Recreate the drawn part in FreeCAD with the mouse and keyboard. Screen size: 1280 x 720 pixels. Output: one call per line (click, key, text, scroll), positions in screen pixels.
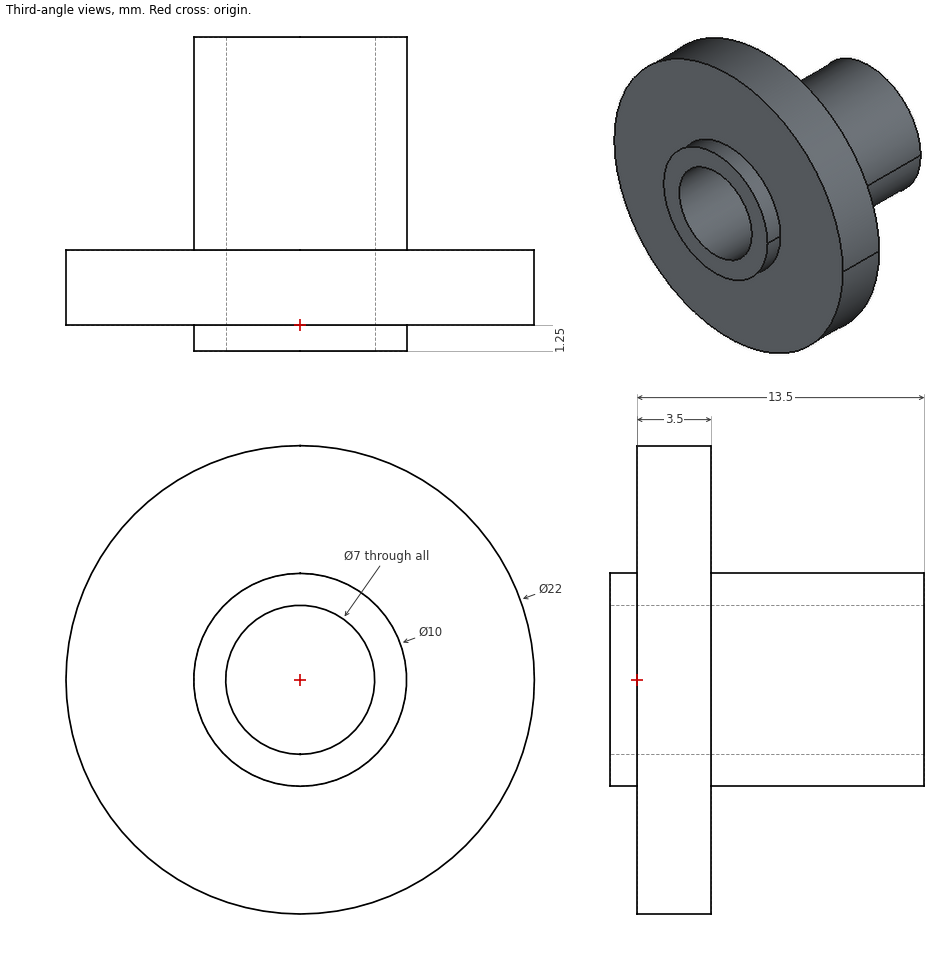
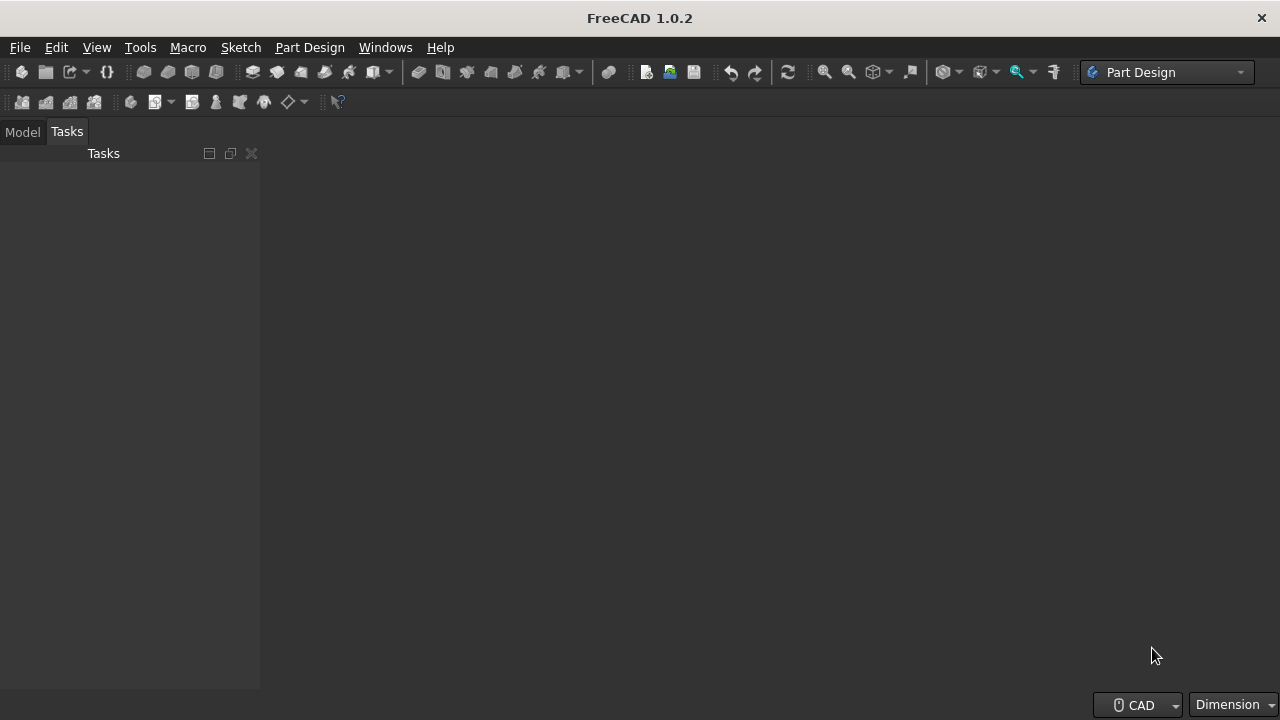
click(646, 72)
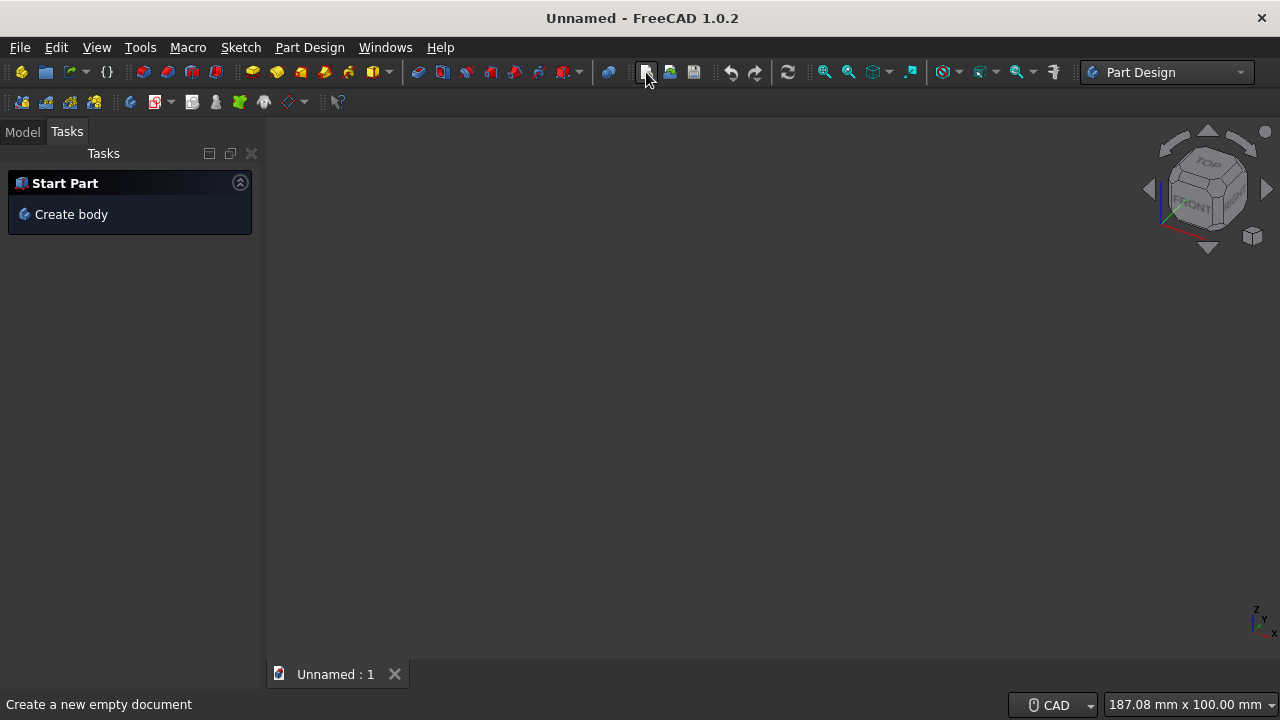
click(156, 102)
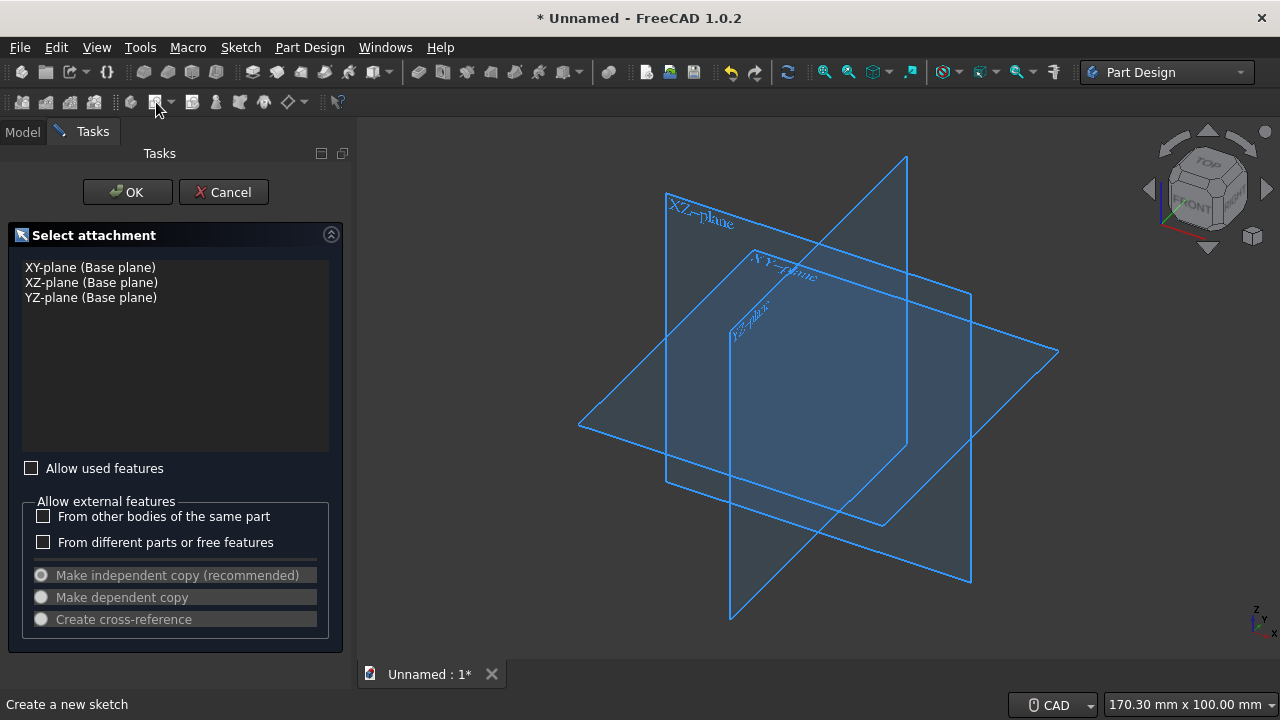
click(82, 282)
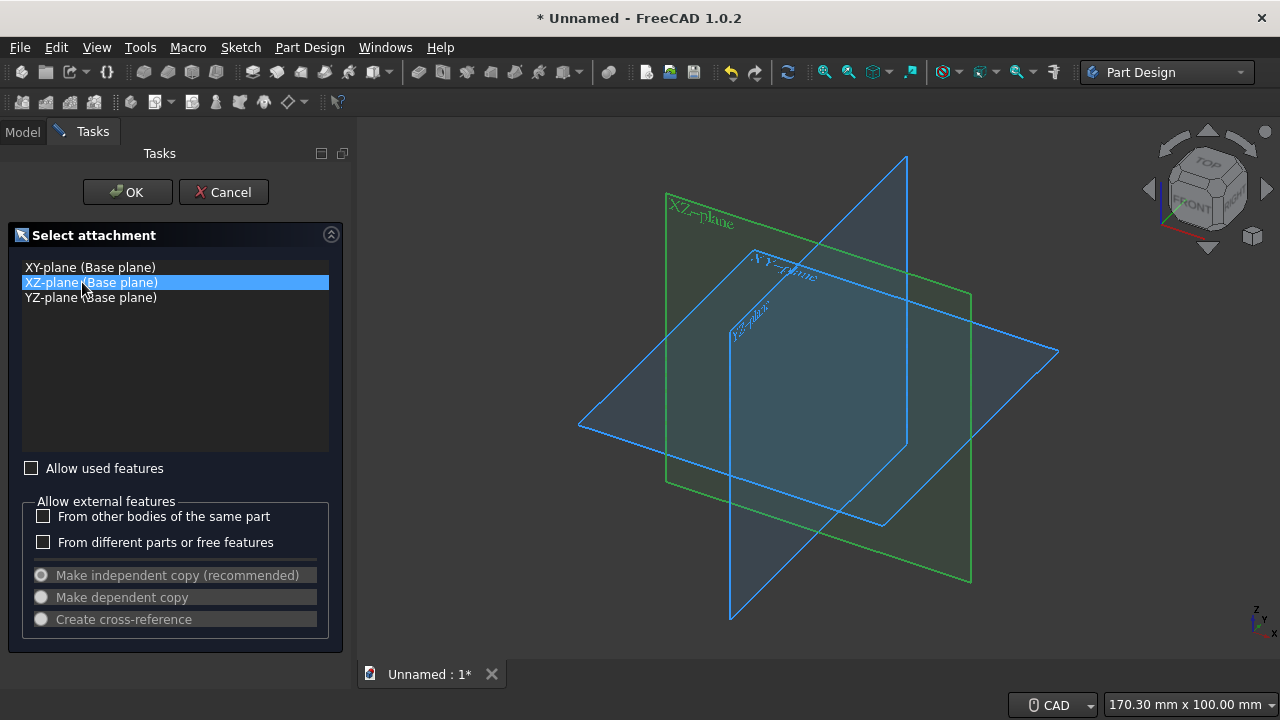
click(128, 192)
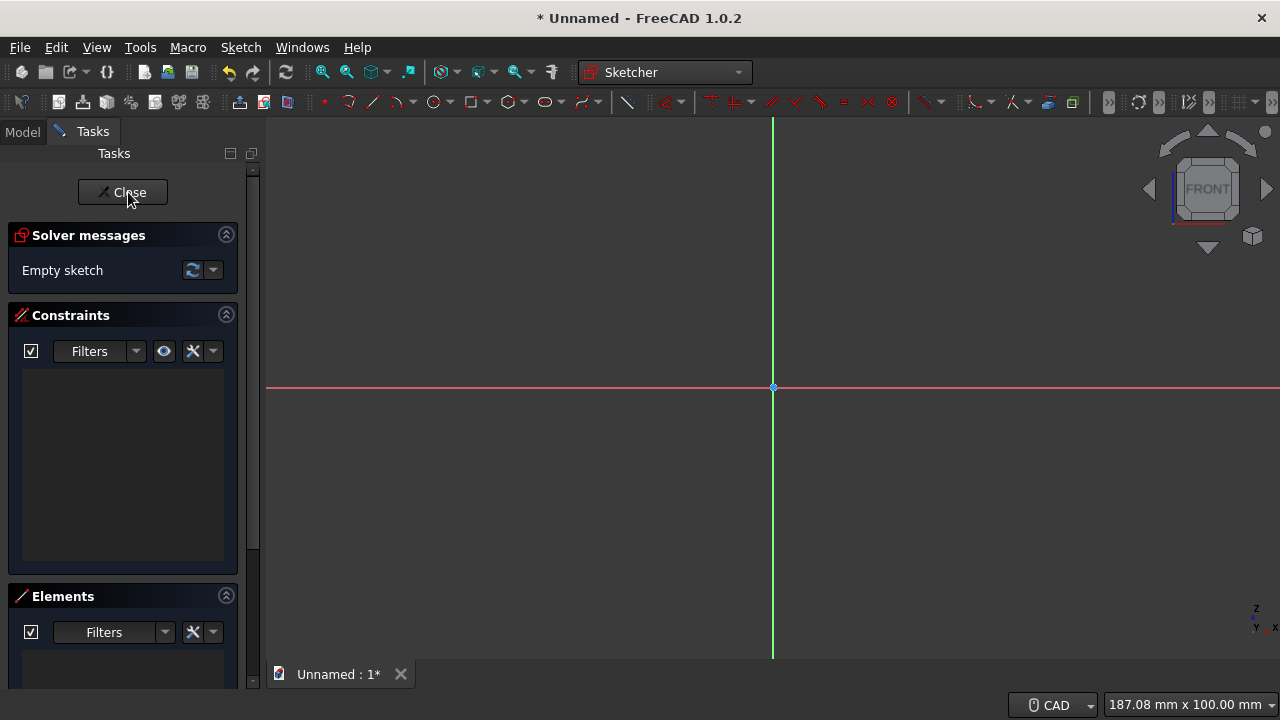
scroll(813, 388, up, 5)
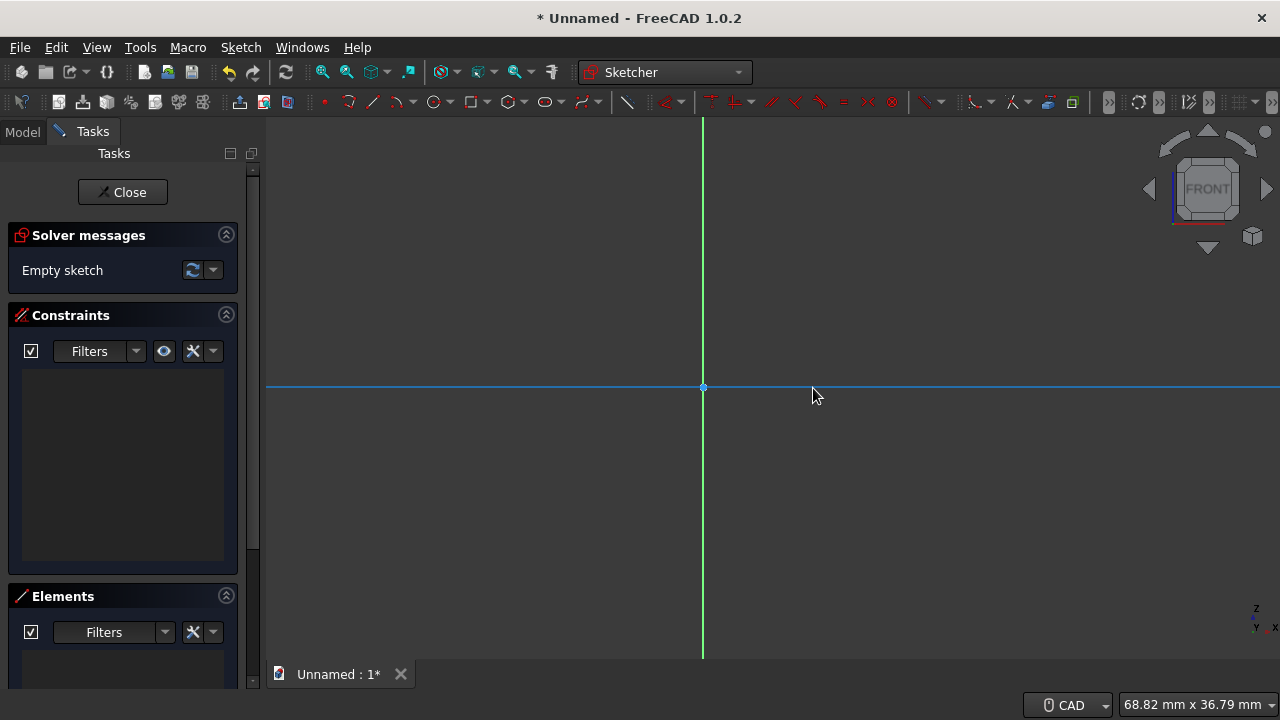
key(g)
key(c)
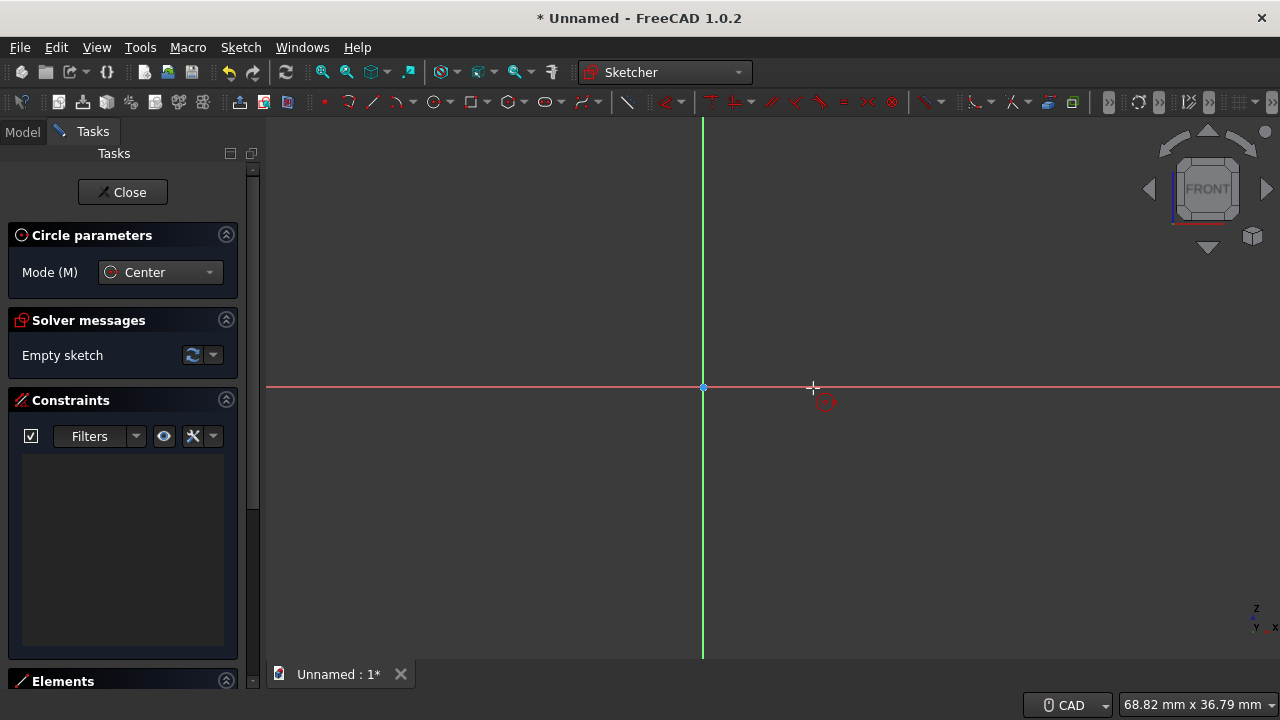
click(703, 387)
move(818, 273)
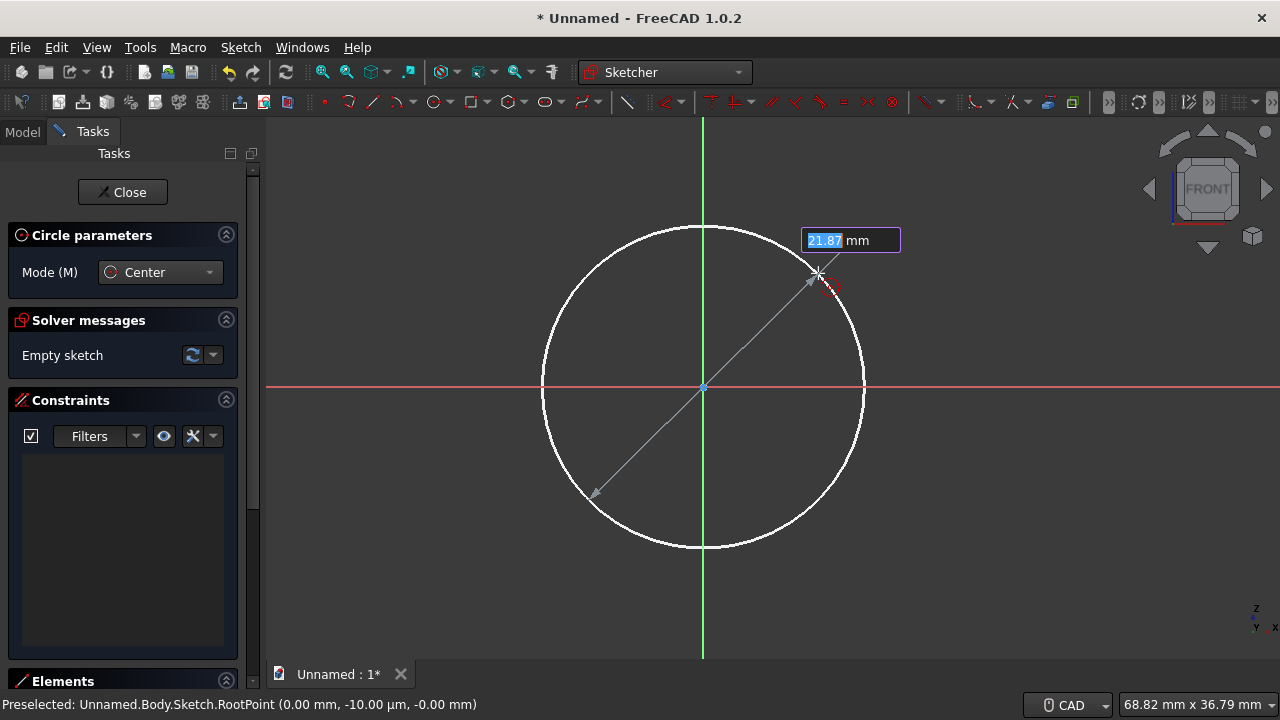
text(22)
key(Return)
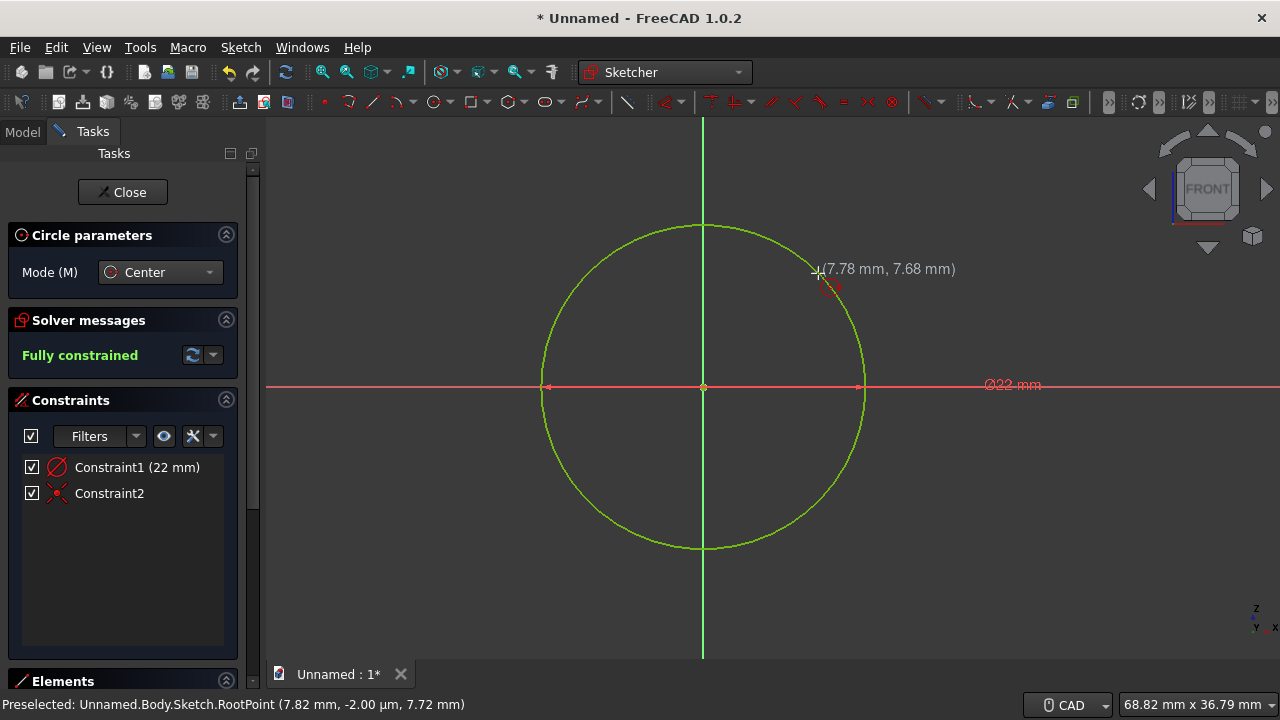
click(703, 387)
move(755, 335)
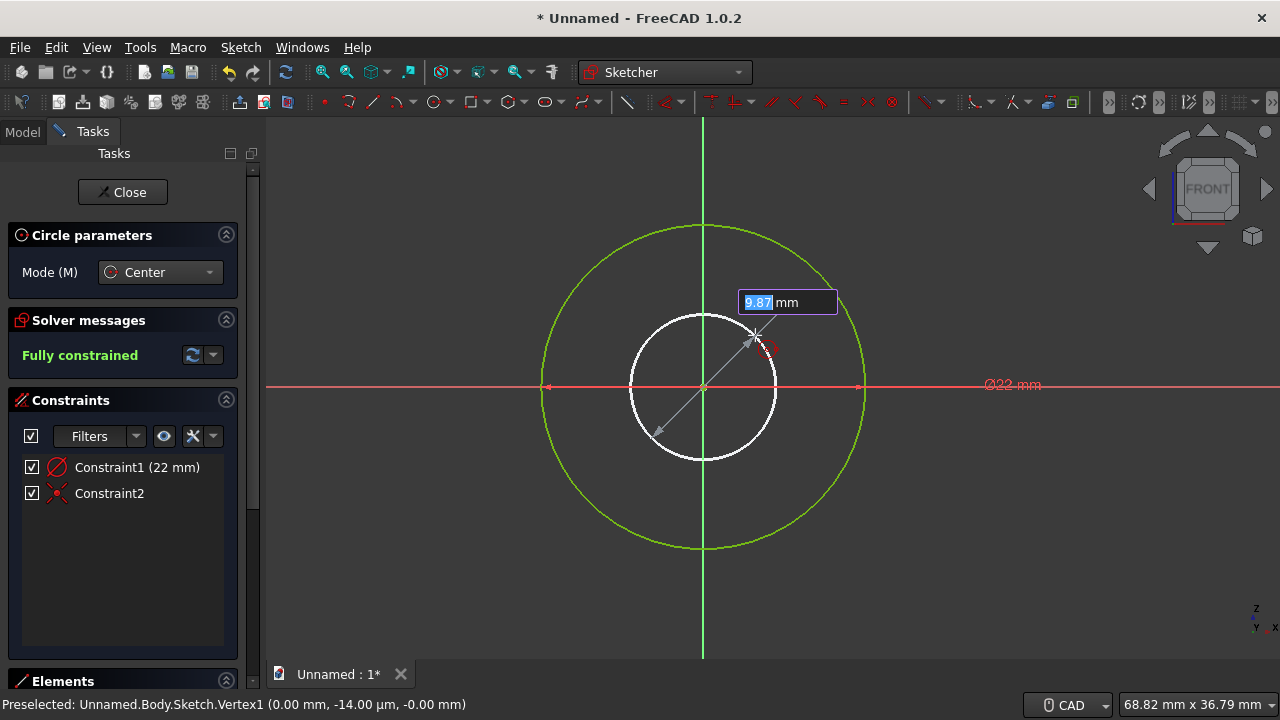
text(10)
key(Return)
key(Escape)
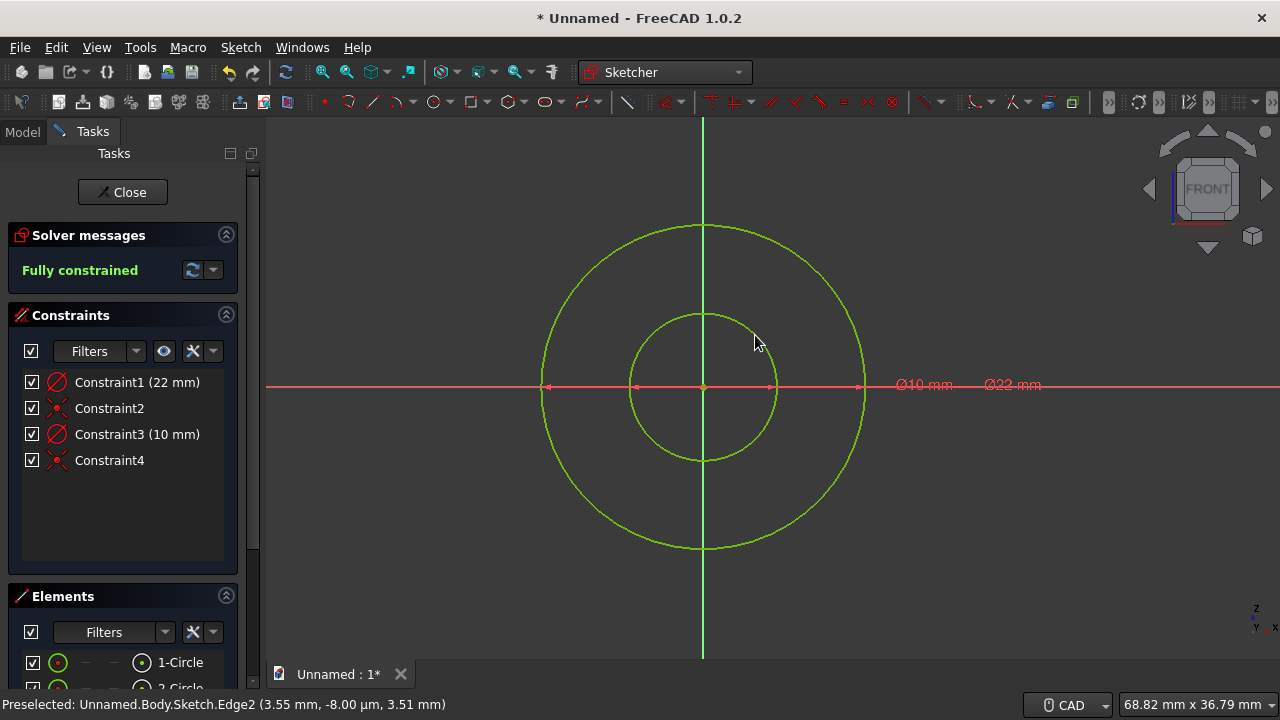
click(123, 192)